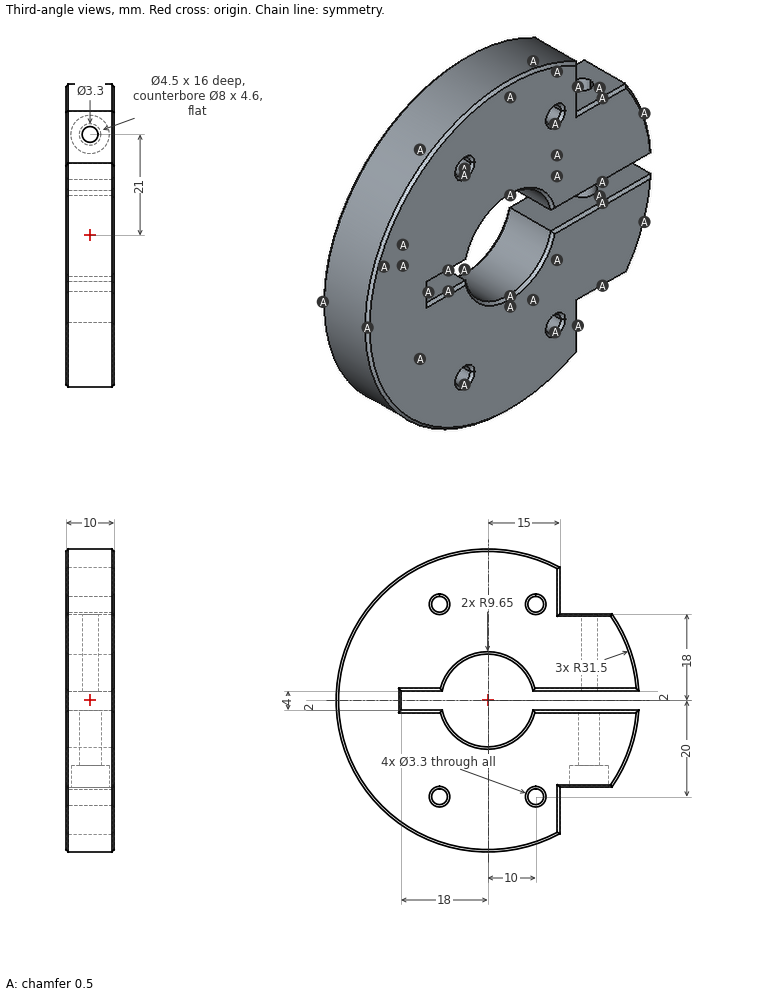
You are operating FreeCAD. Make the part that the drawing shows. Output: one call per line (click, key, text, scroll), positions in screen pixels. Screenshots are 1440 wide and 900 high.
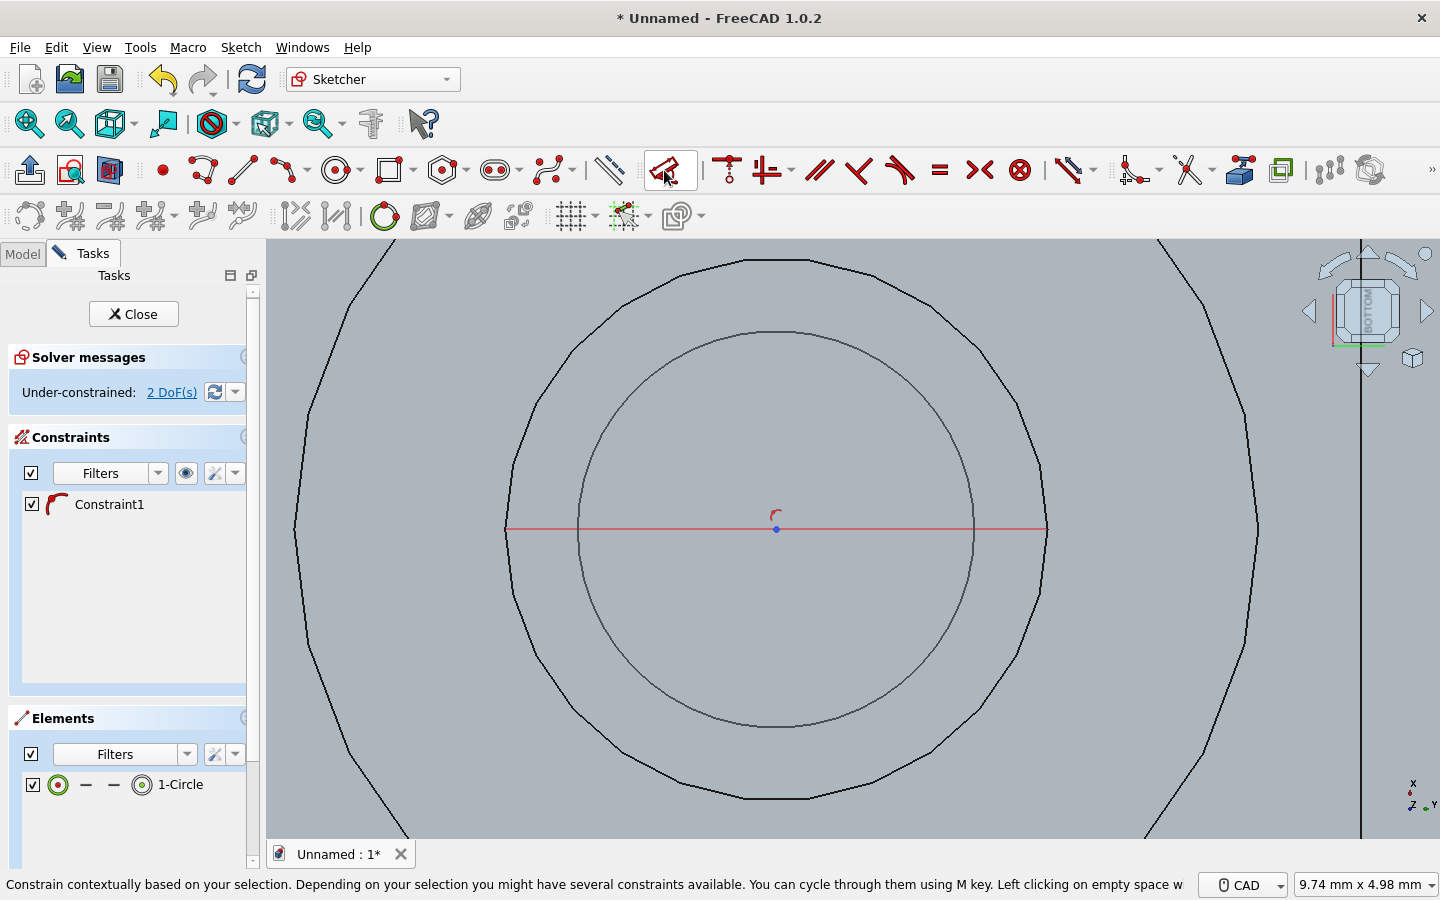
click(916, 389)
click(939, 366)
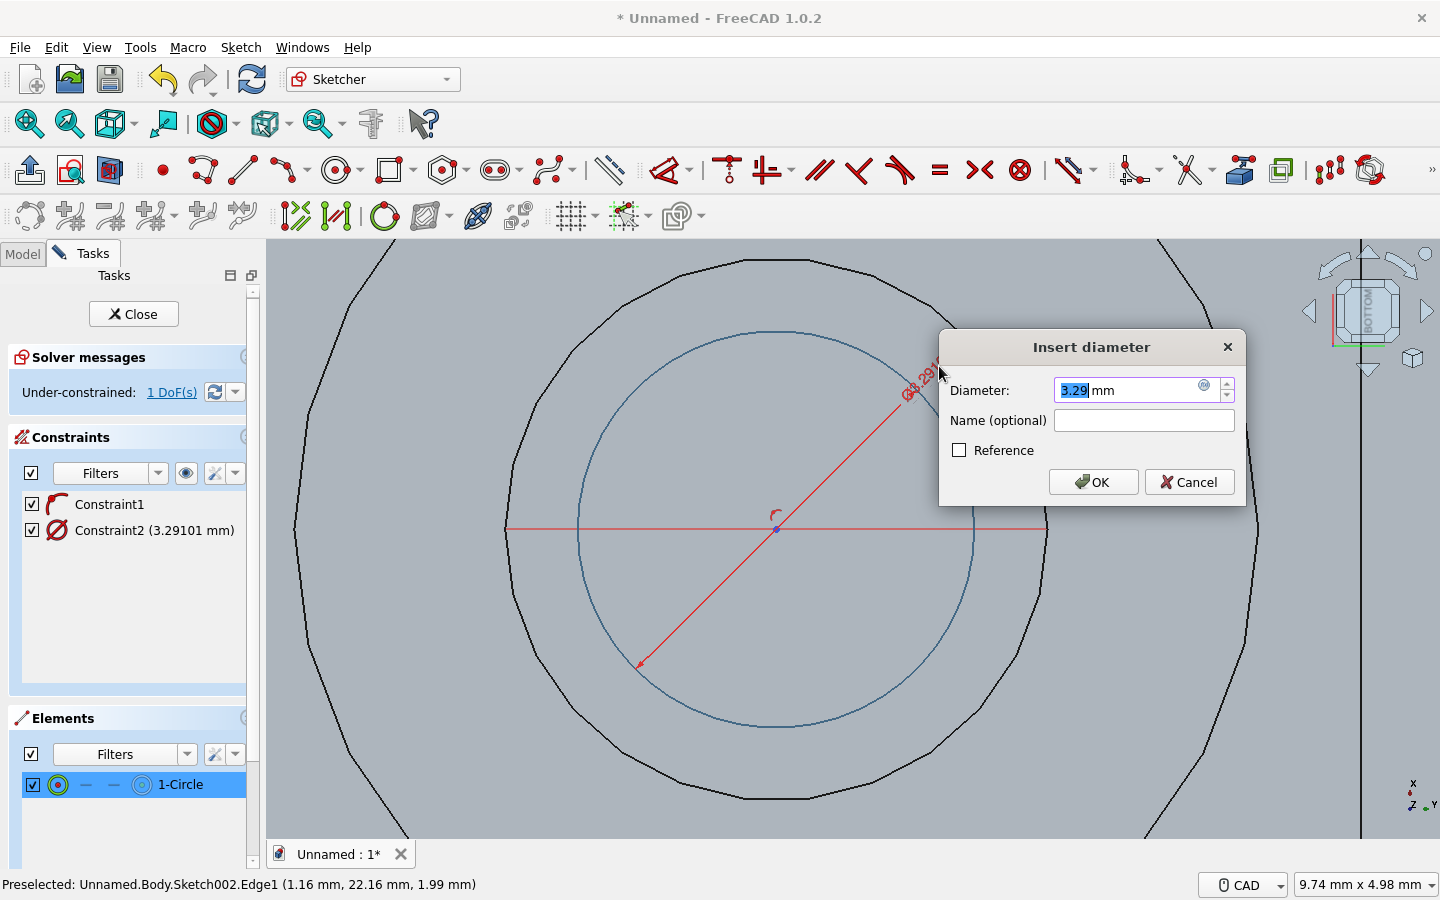
text(3.3)
key(Return)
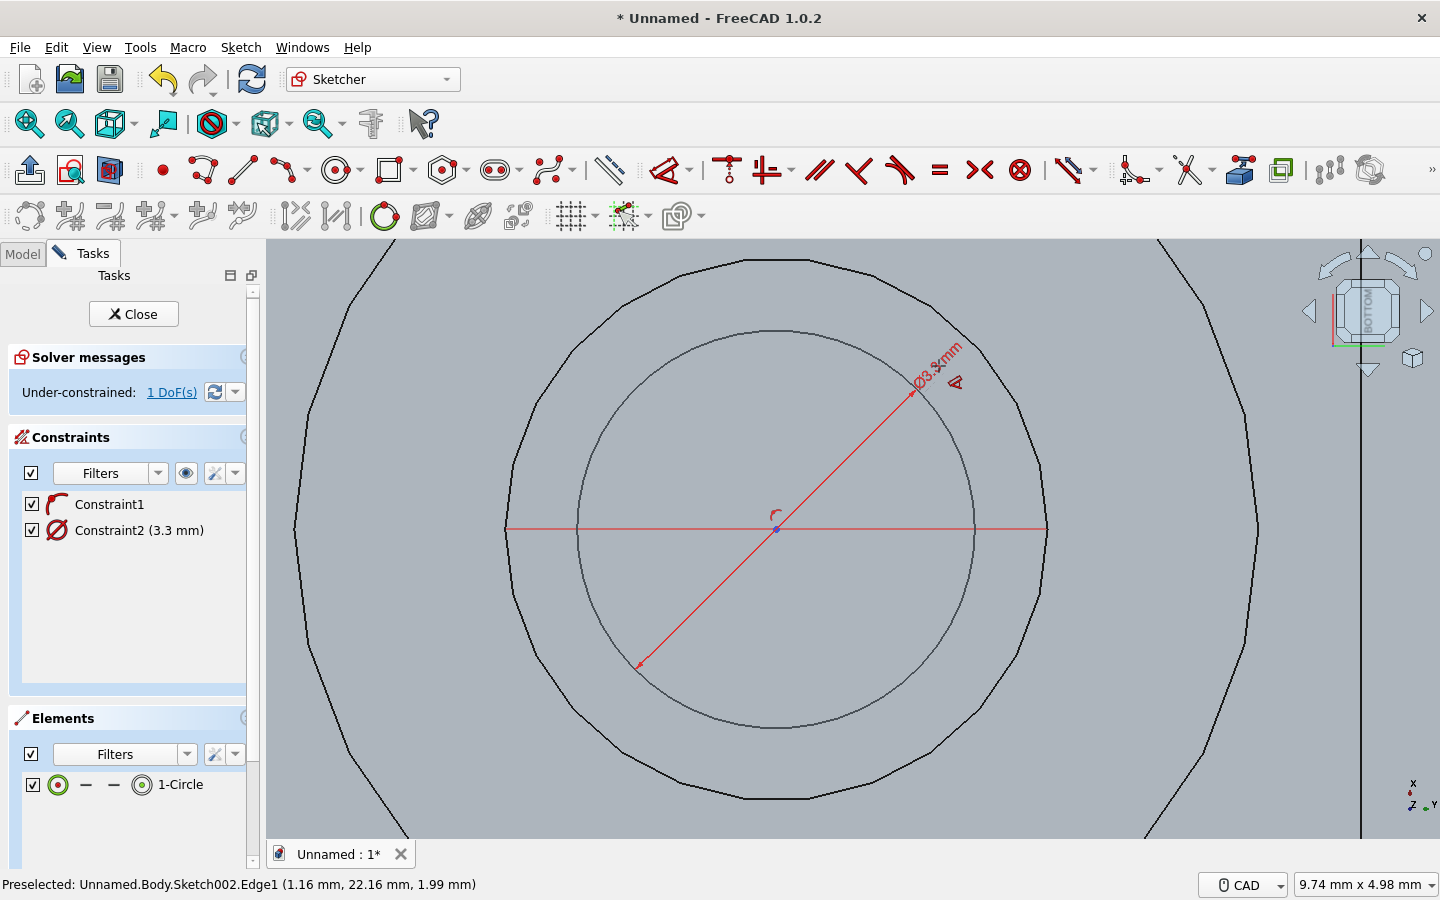
click(776, 529)
click(535, 563)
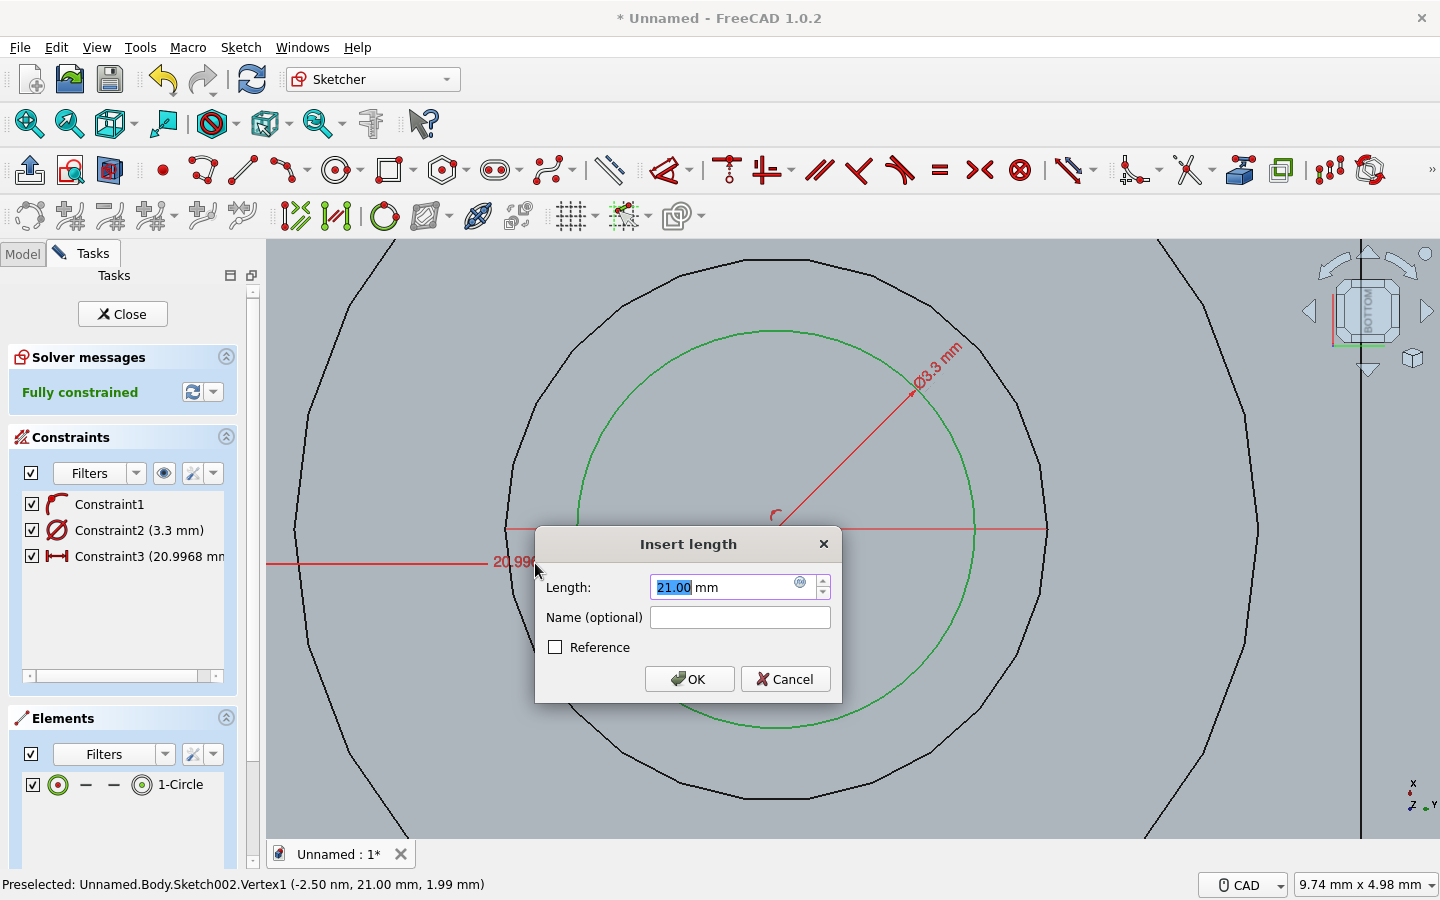
text(21)
key(Return)
key(Escape)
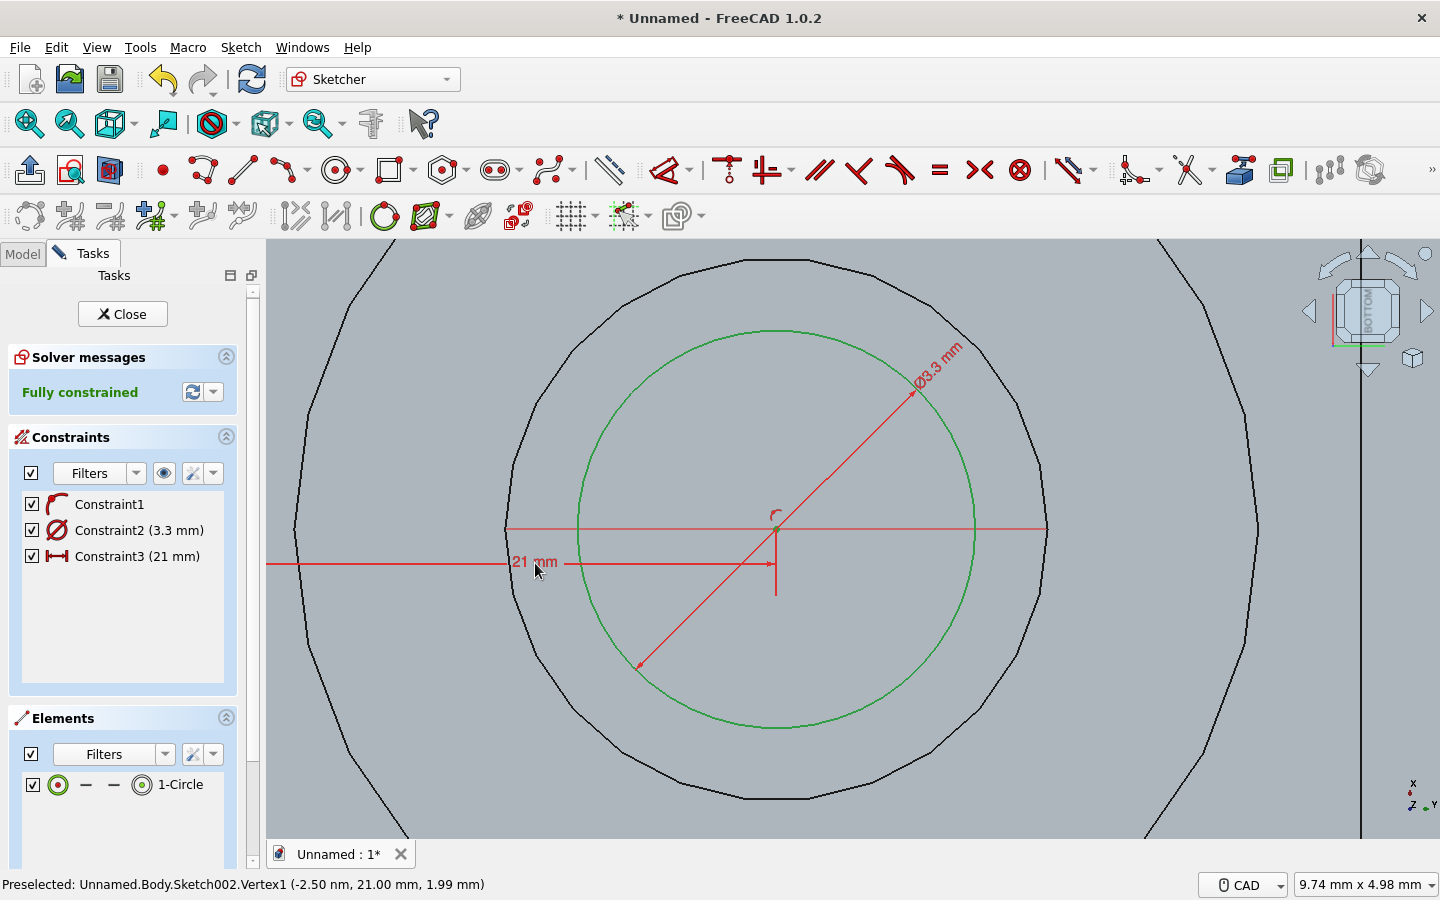
click(123, 314)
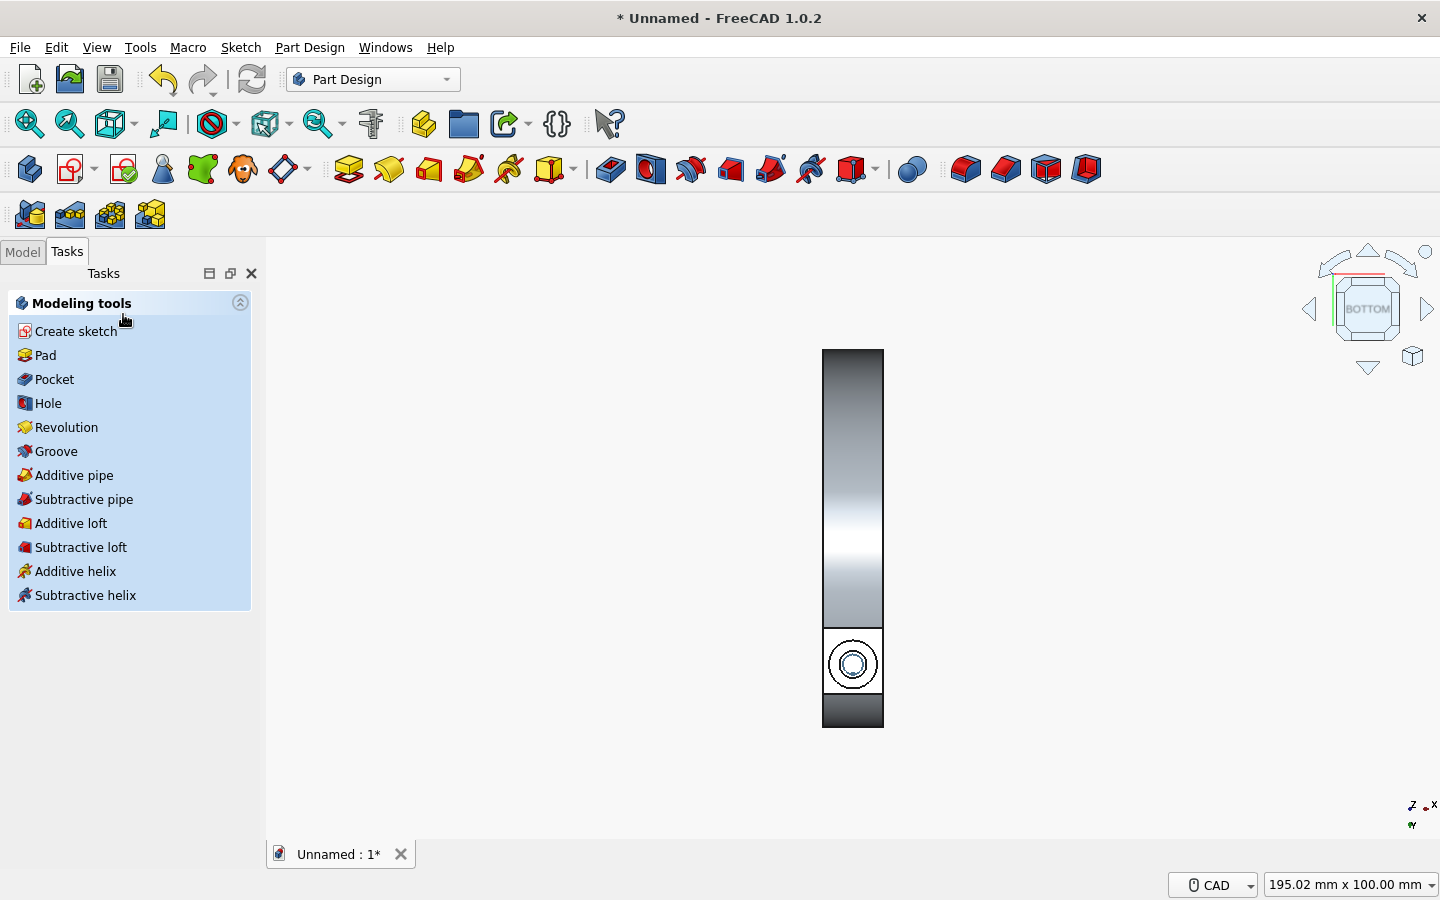
click(612, 170)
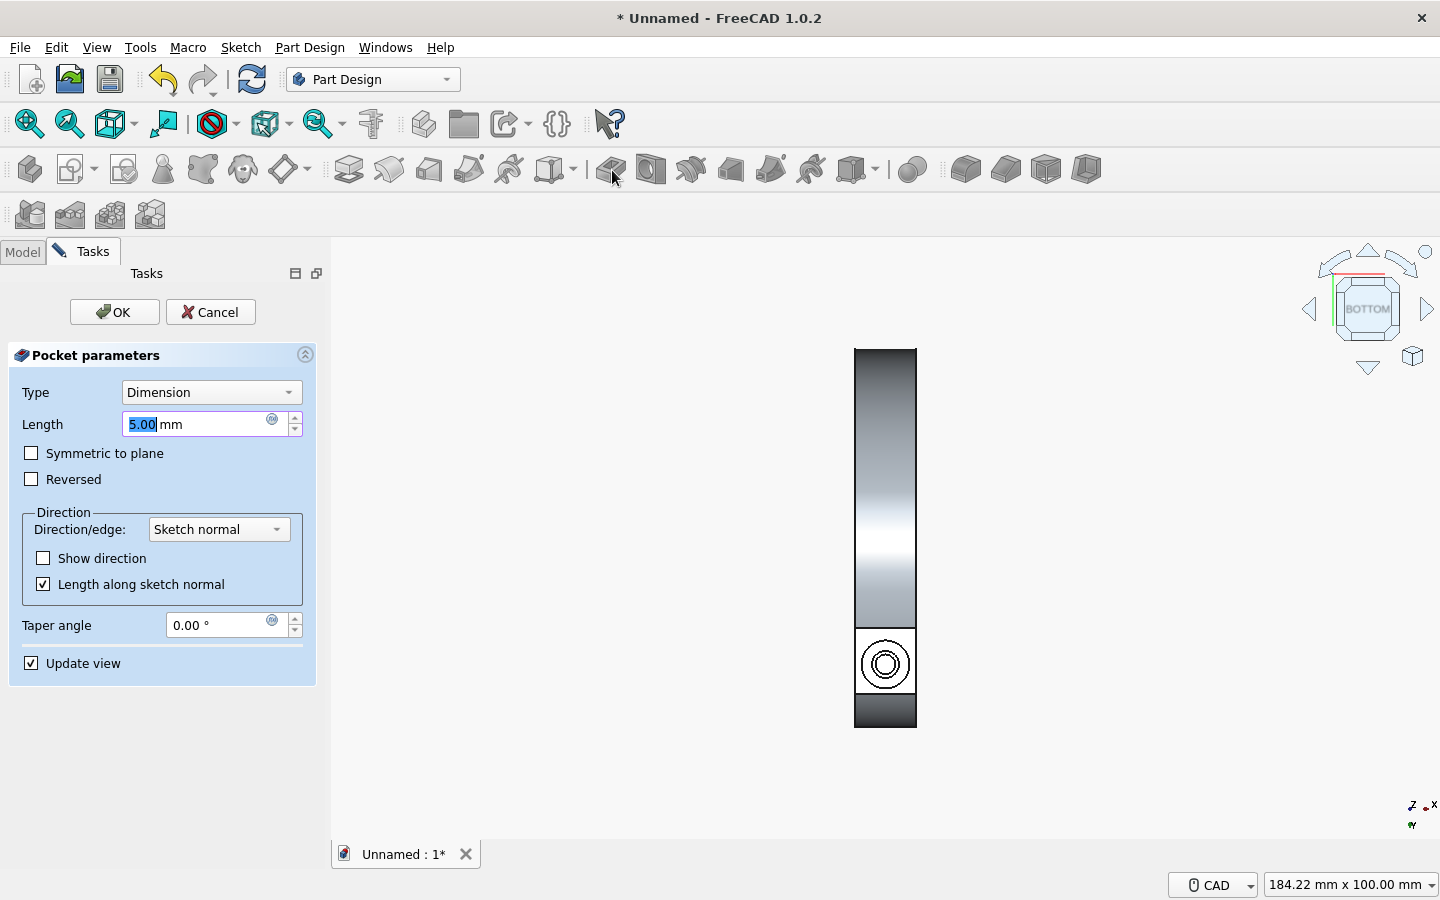
click(212, 392)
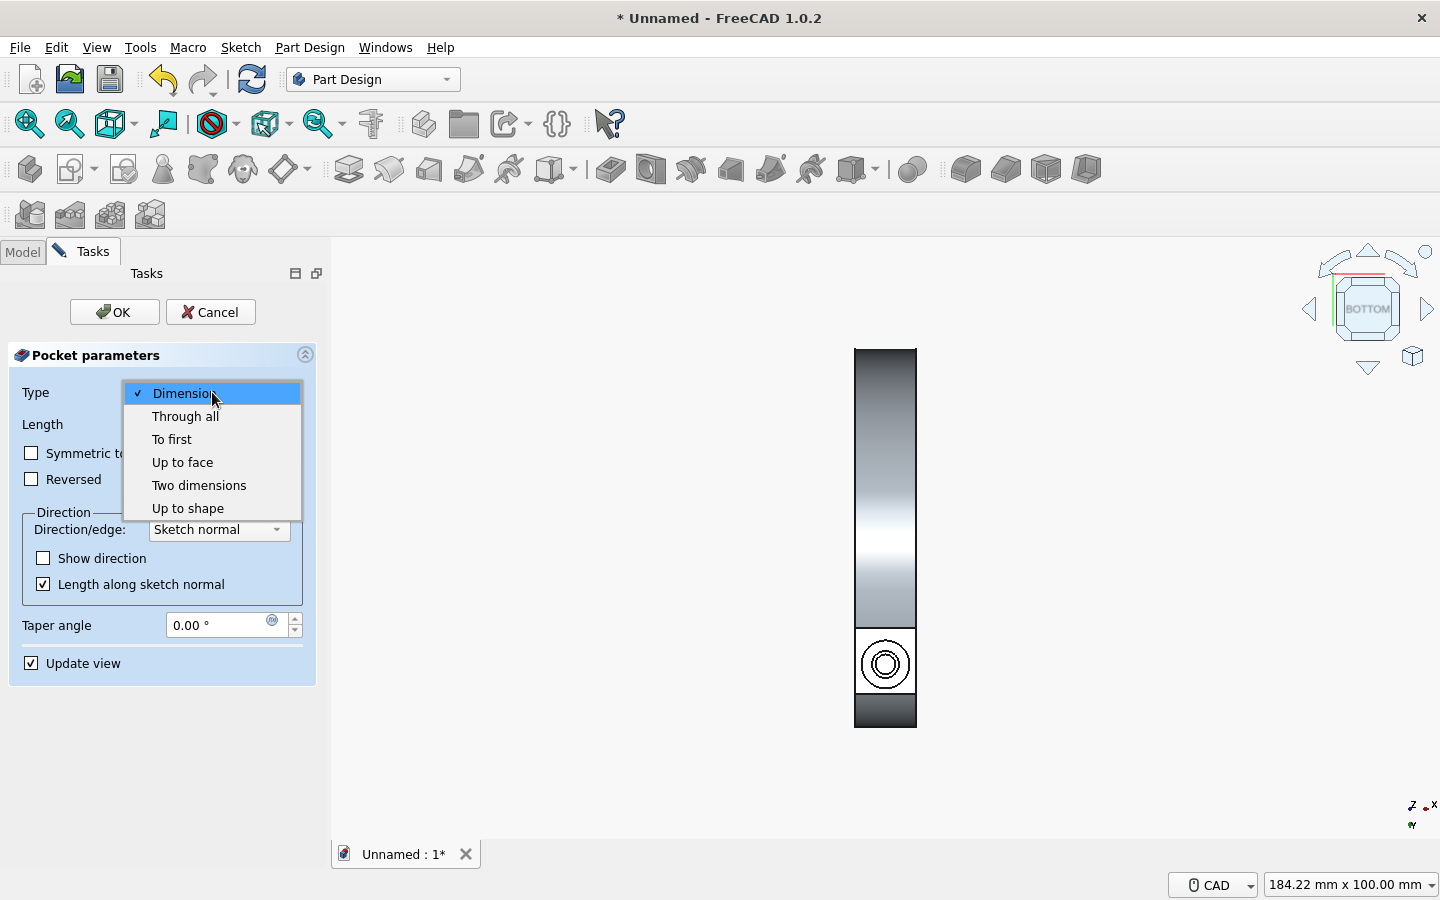
click(212, 416)